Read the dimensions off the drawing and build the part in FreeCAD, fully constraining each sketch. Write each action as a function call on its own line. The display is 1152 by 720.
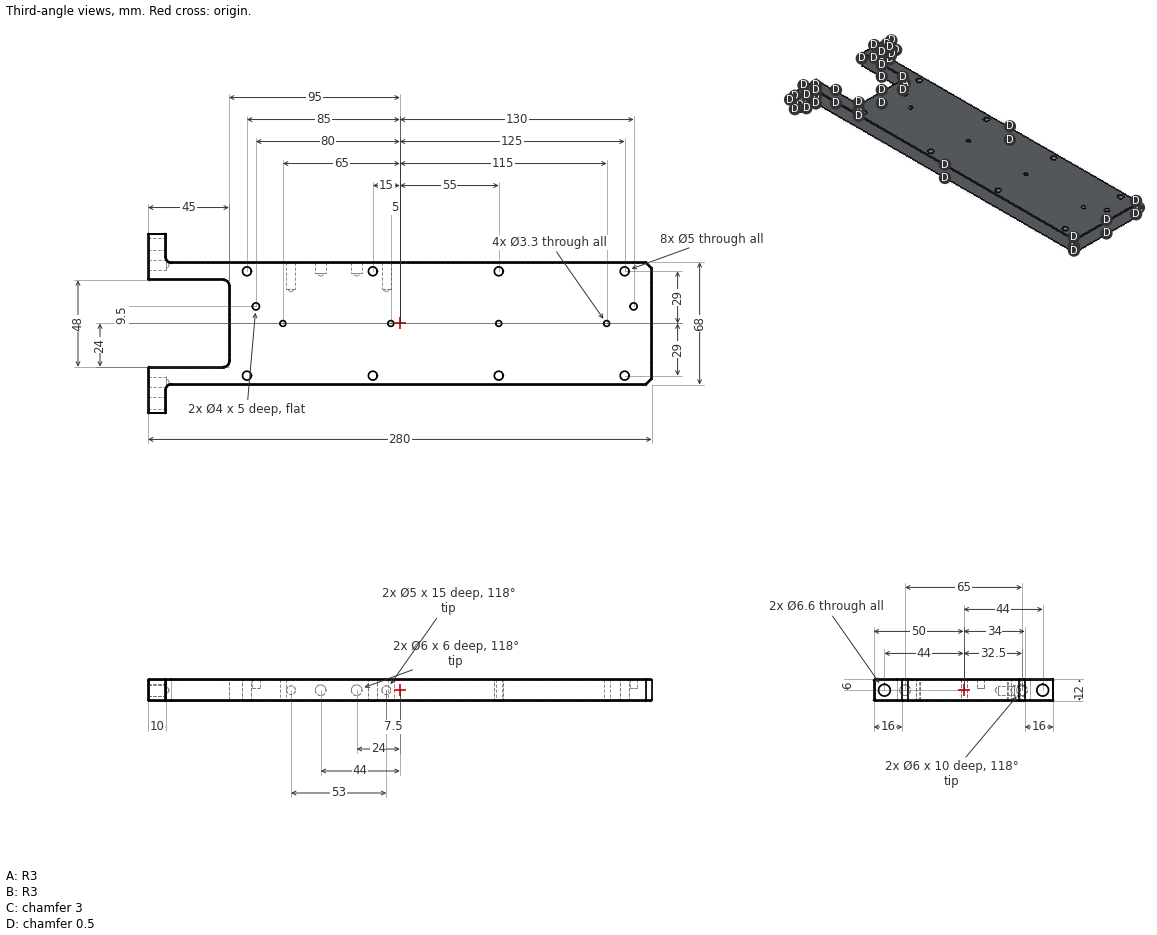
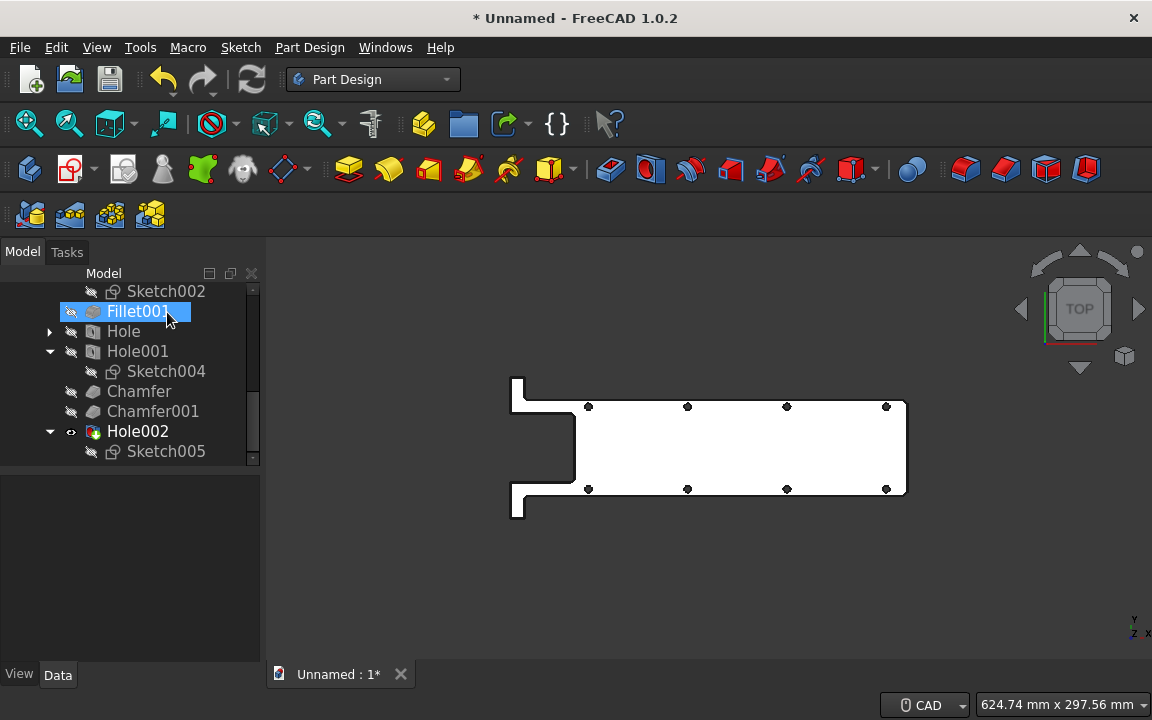
key(v)
key(f)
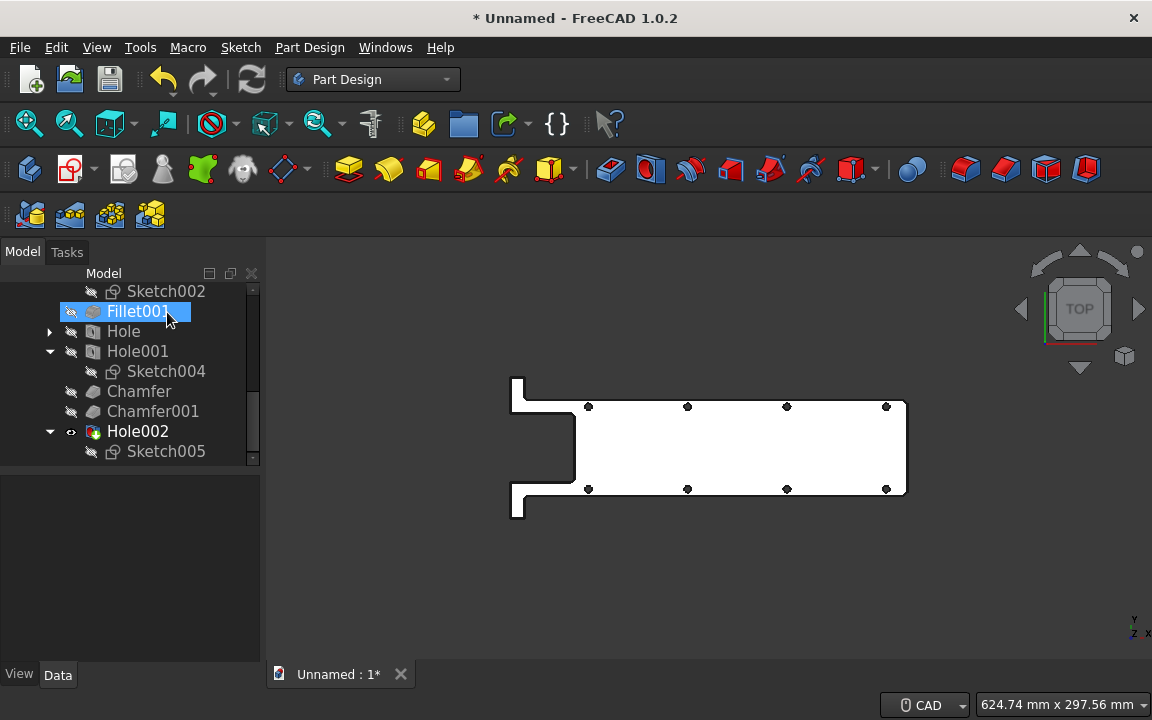
key(3)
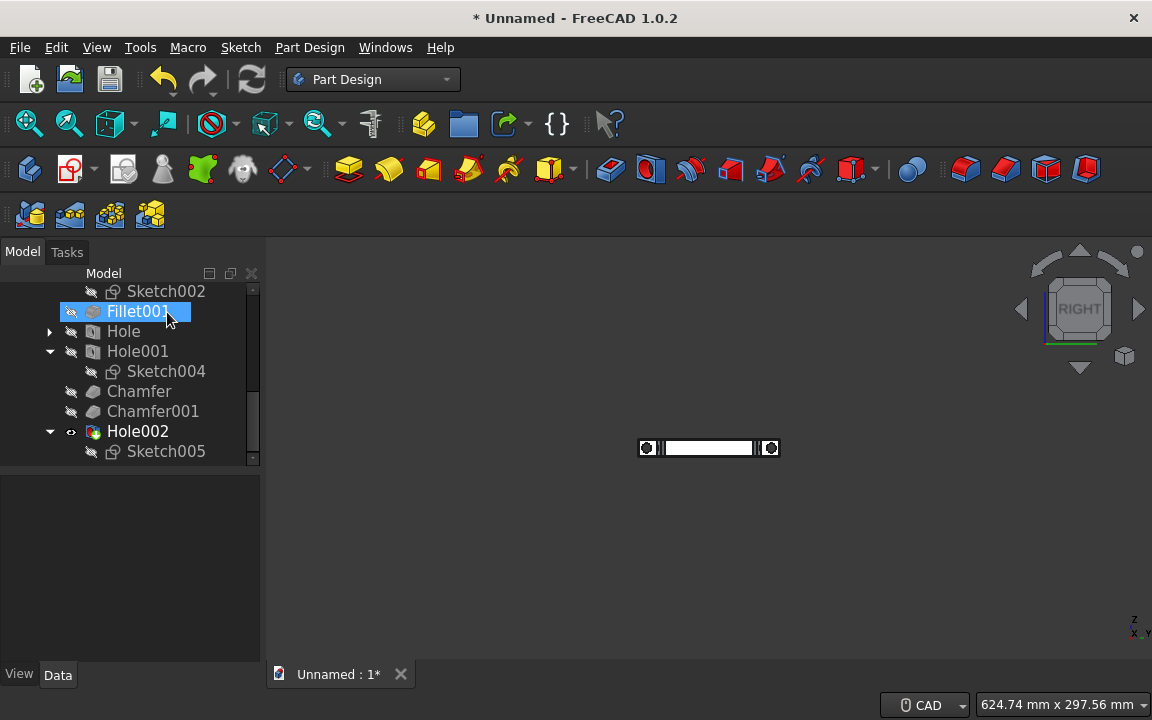
key(v)
key(f)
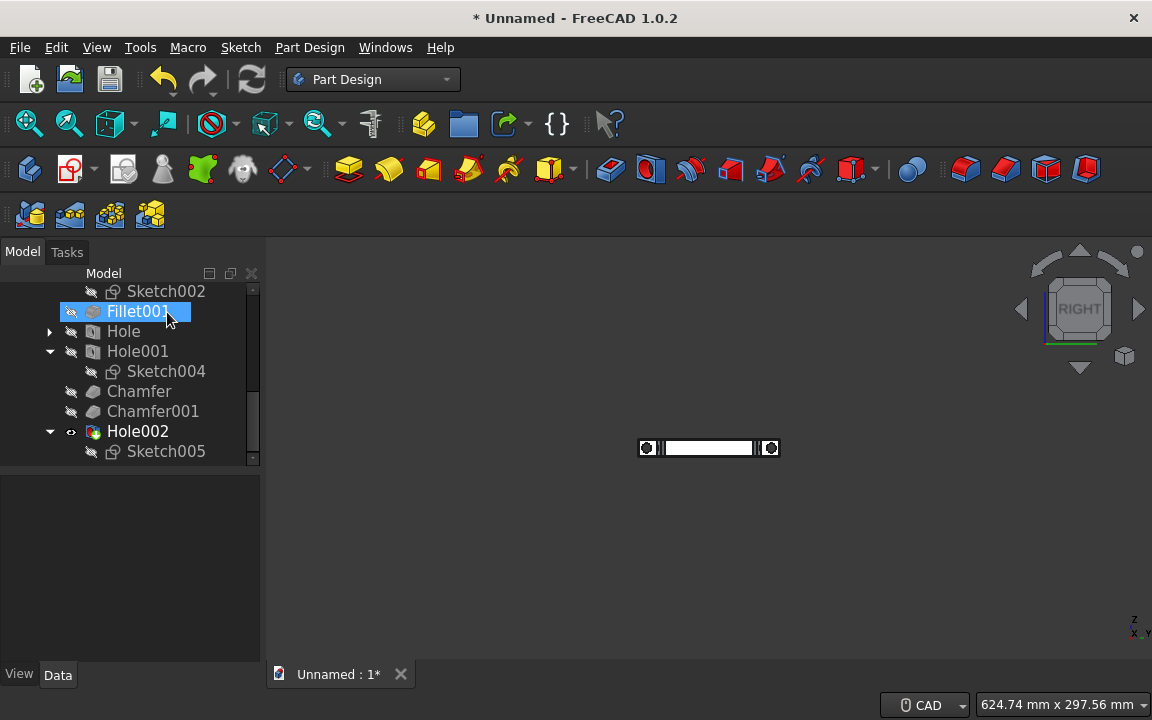
scroll(160, 367, down, 3)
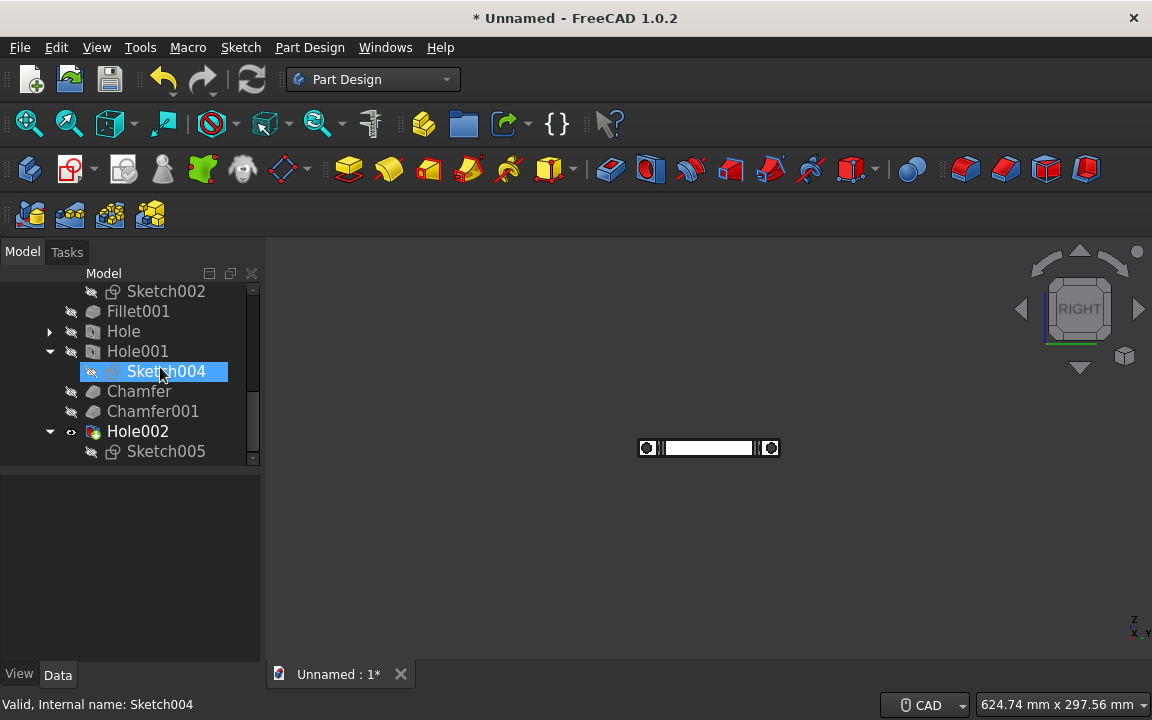
scroll(160, 367, up, 15)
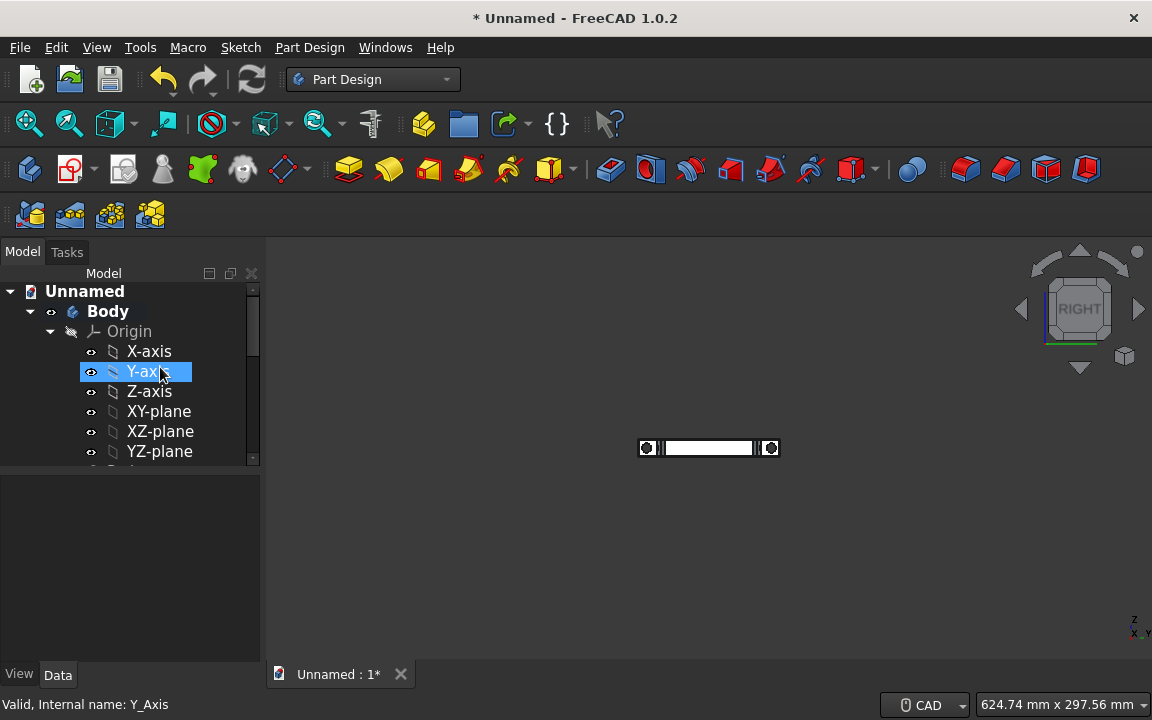
click(136, 432)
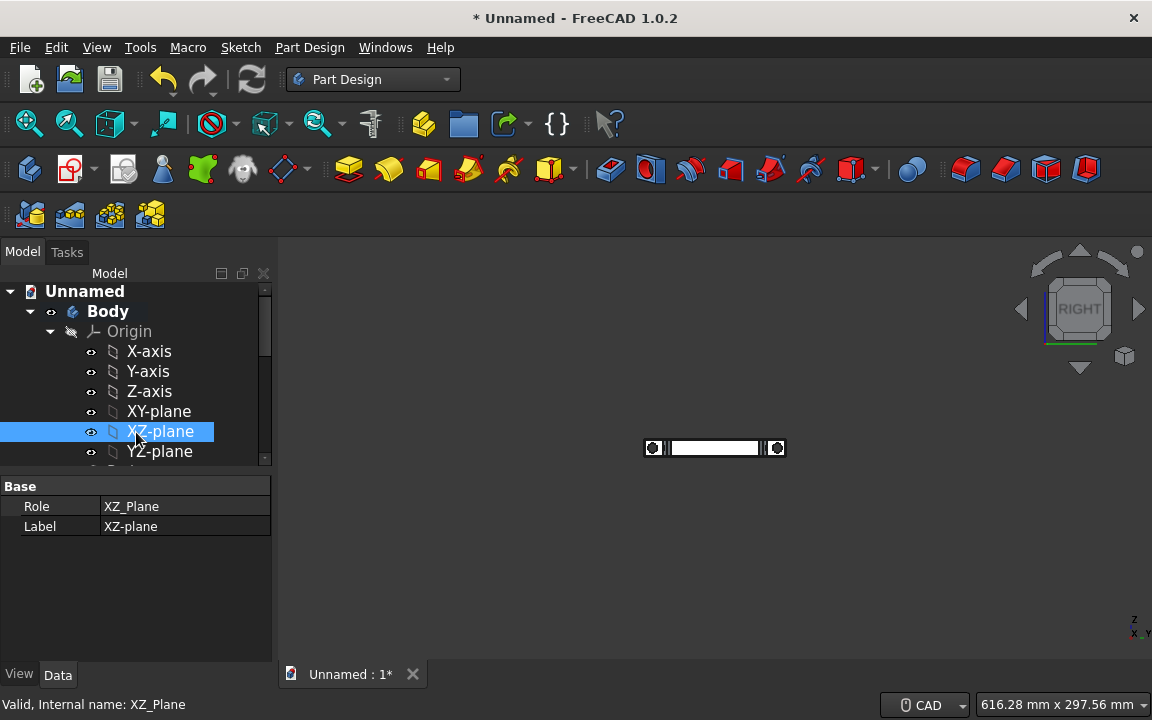
click(284, 170)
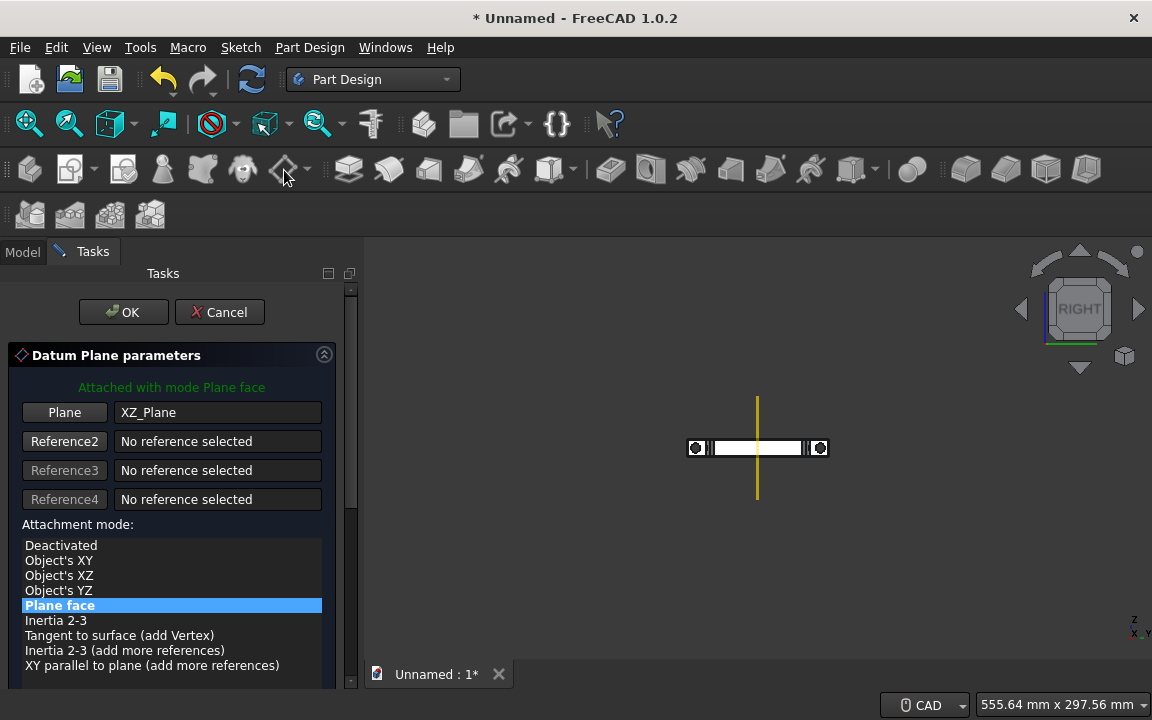
scroll(351, 486, down, 4)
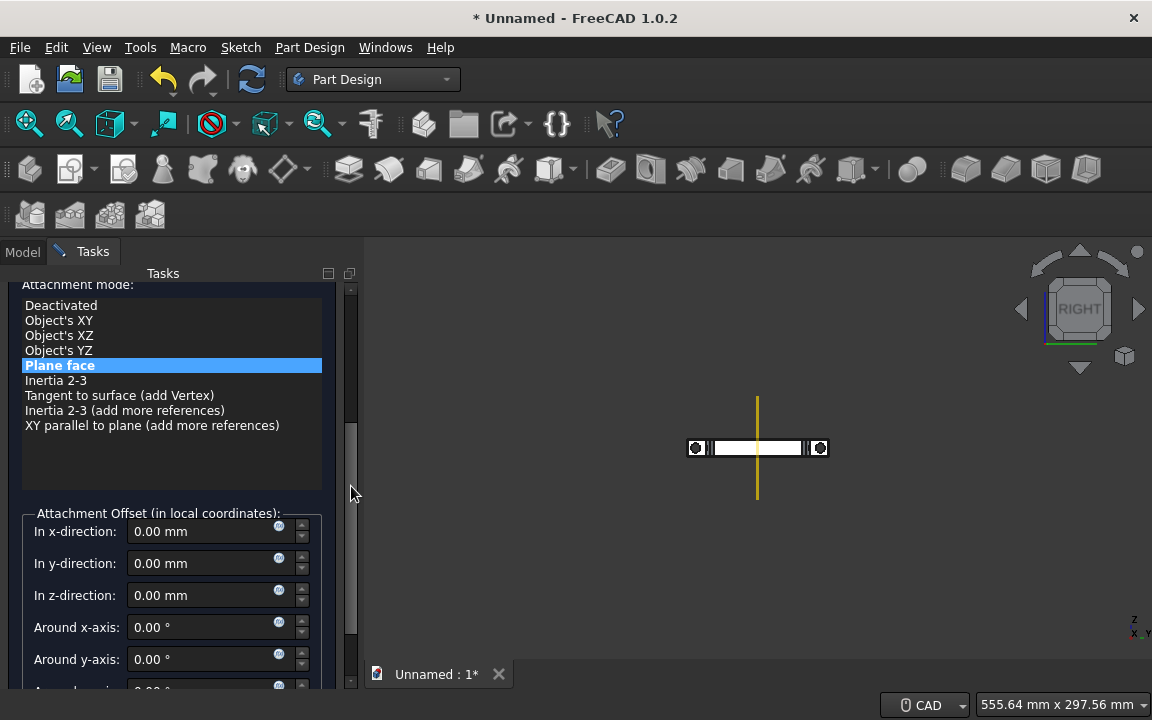
triple_click(210, 595)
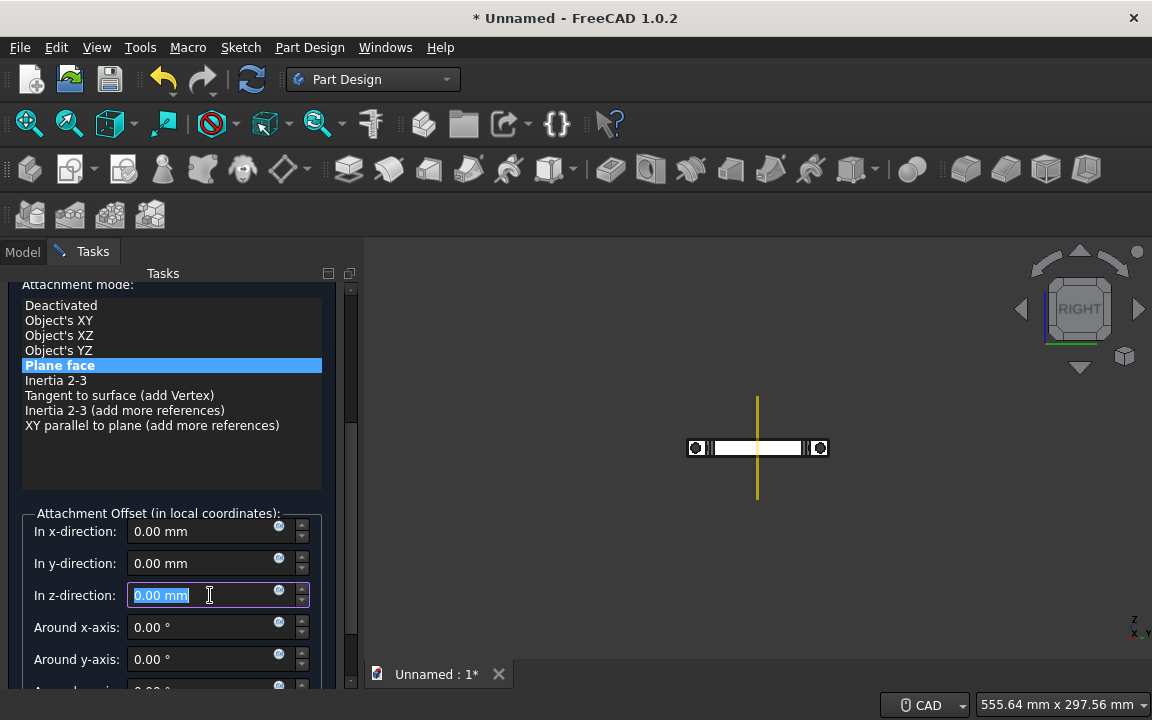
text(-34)
key(Tab)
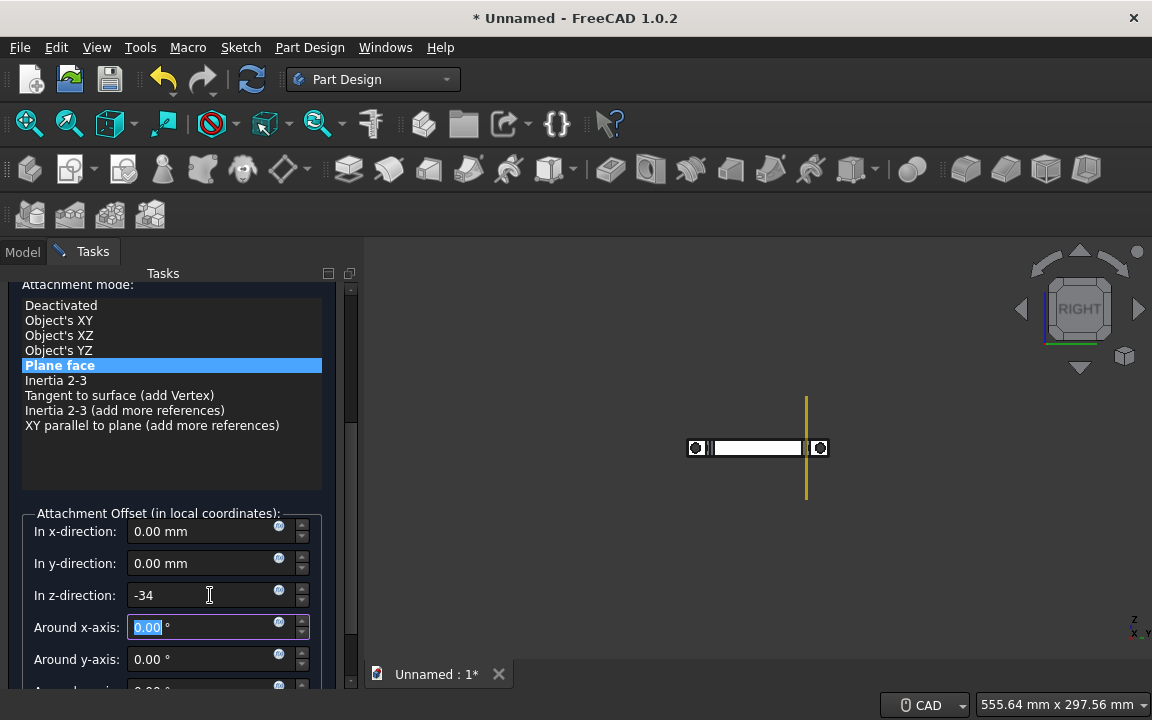
scroll(351, 486, up, 5)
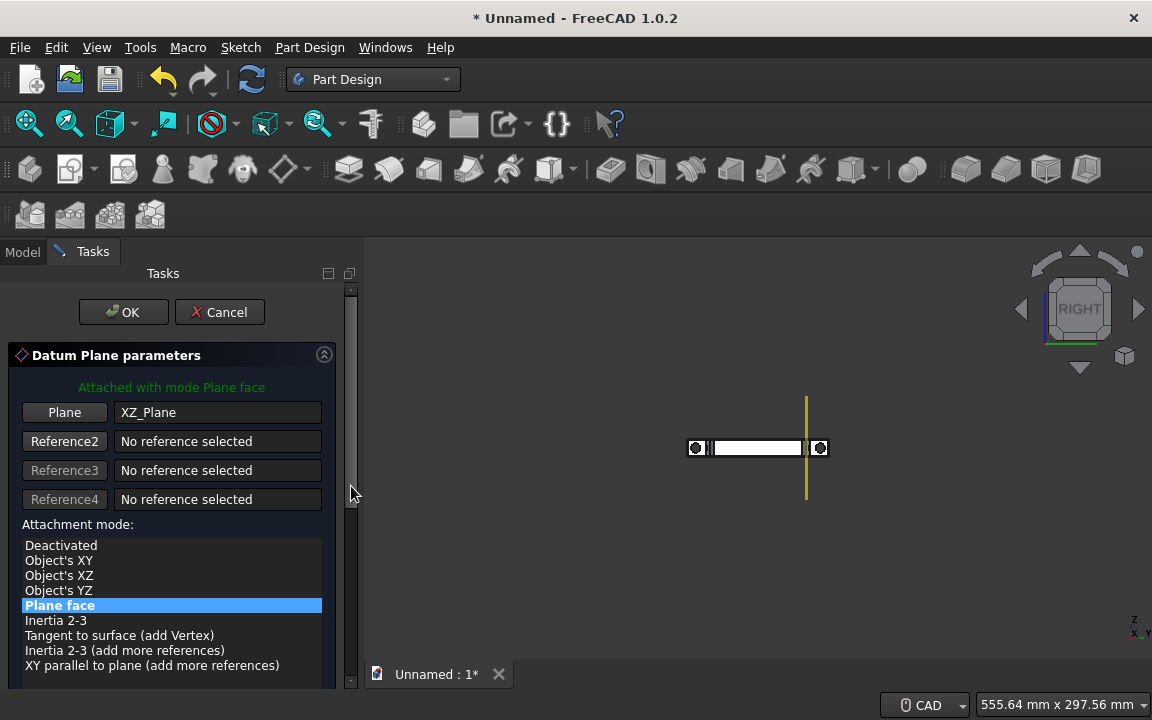
click(124, 312)